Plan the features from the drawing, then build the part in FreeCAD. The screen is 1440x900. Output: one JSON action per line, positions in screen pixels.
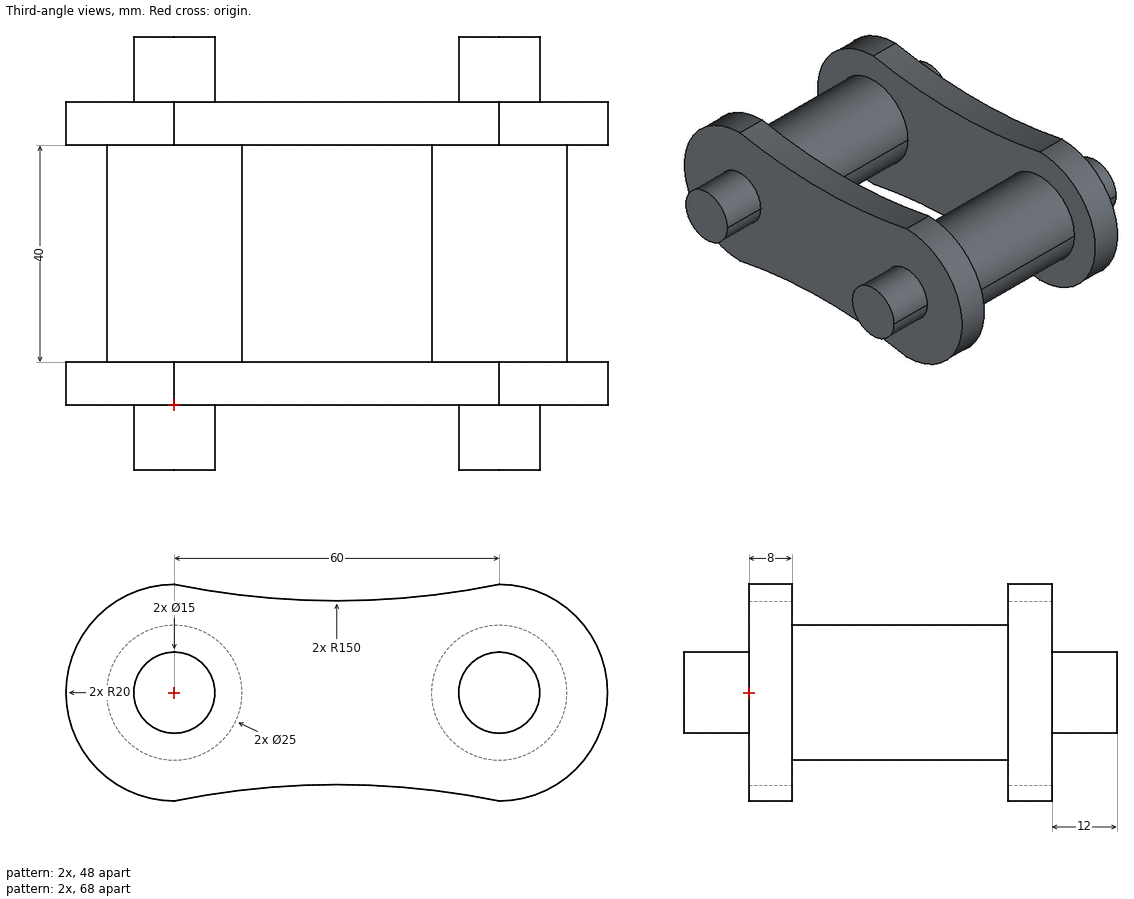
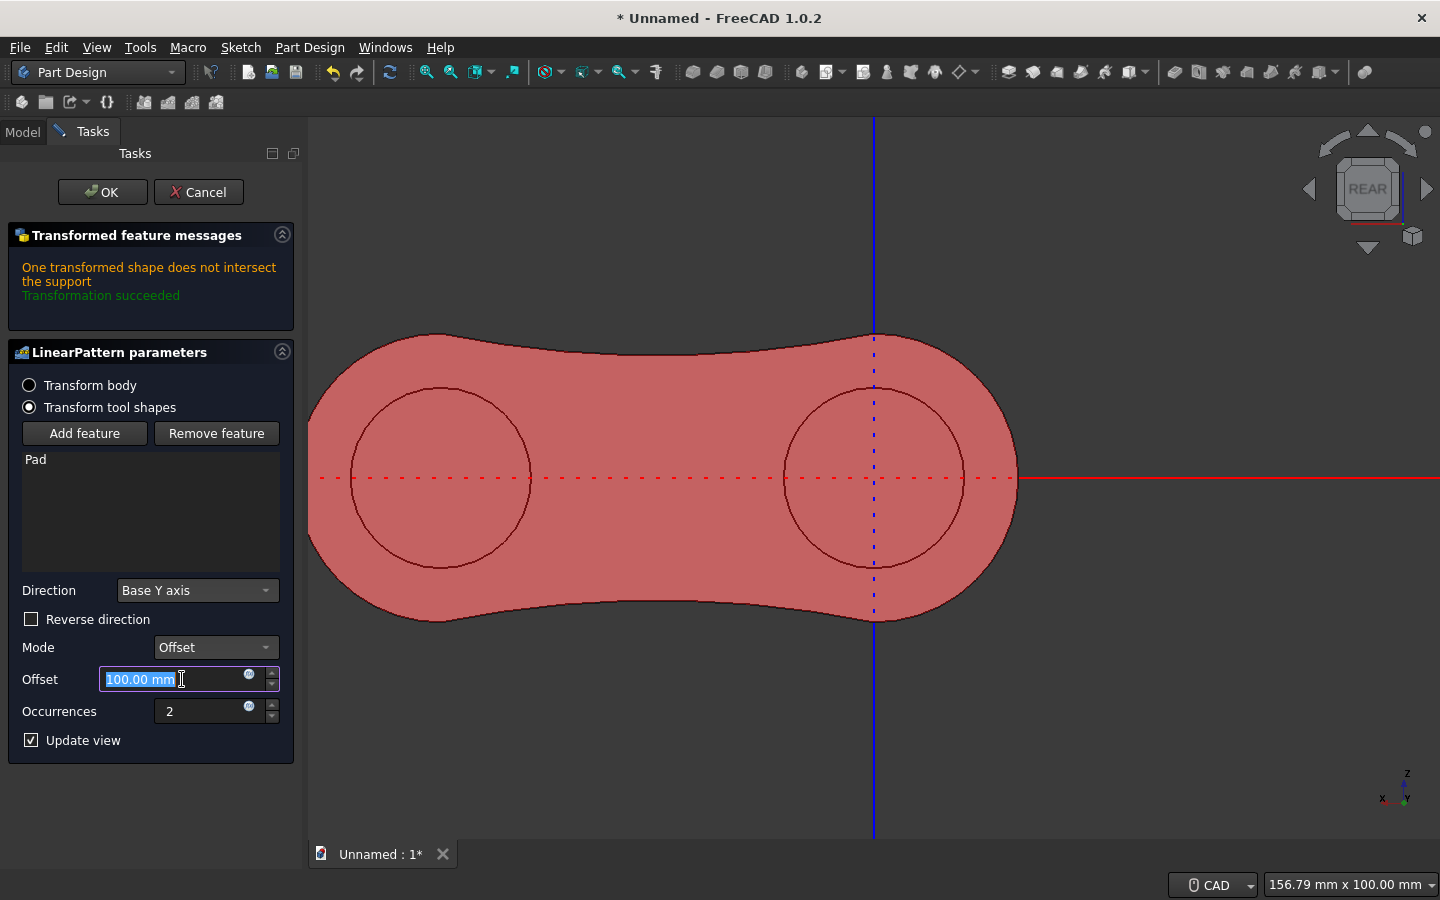
{"action": "type", "text": "48"}
{"action": "key", "text": "Tab"}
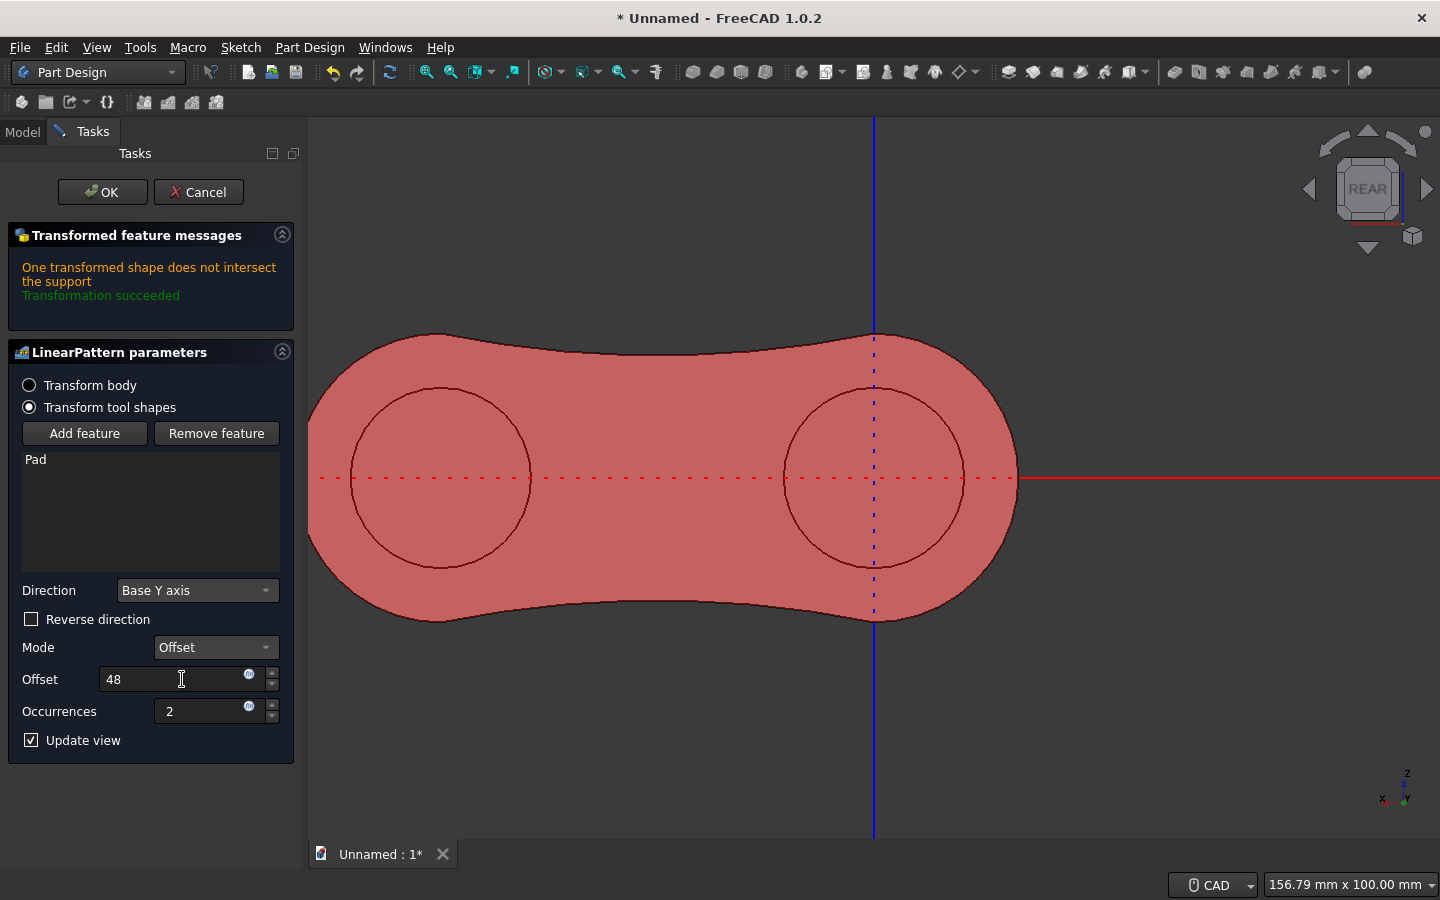
{"action": "triple_click", "coordinate": [209, 711]}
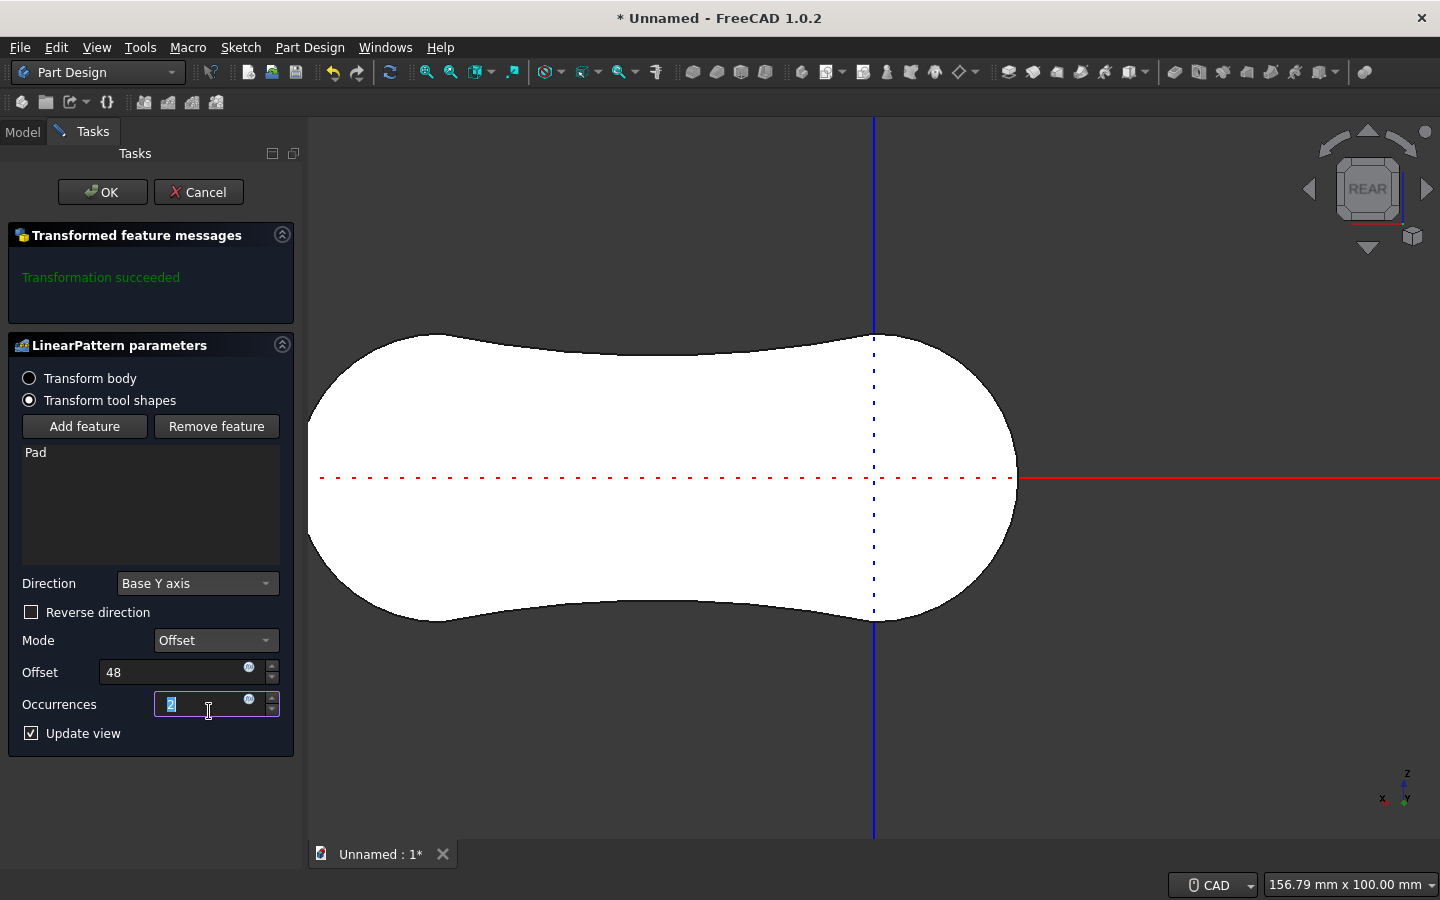
{"action": "type", "text": "2"}
{"action": "key", "text": "Tab"}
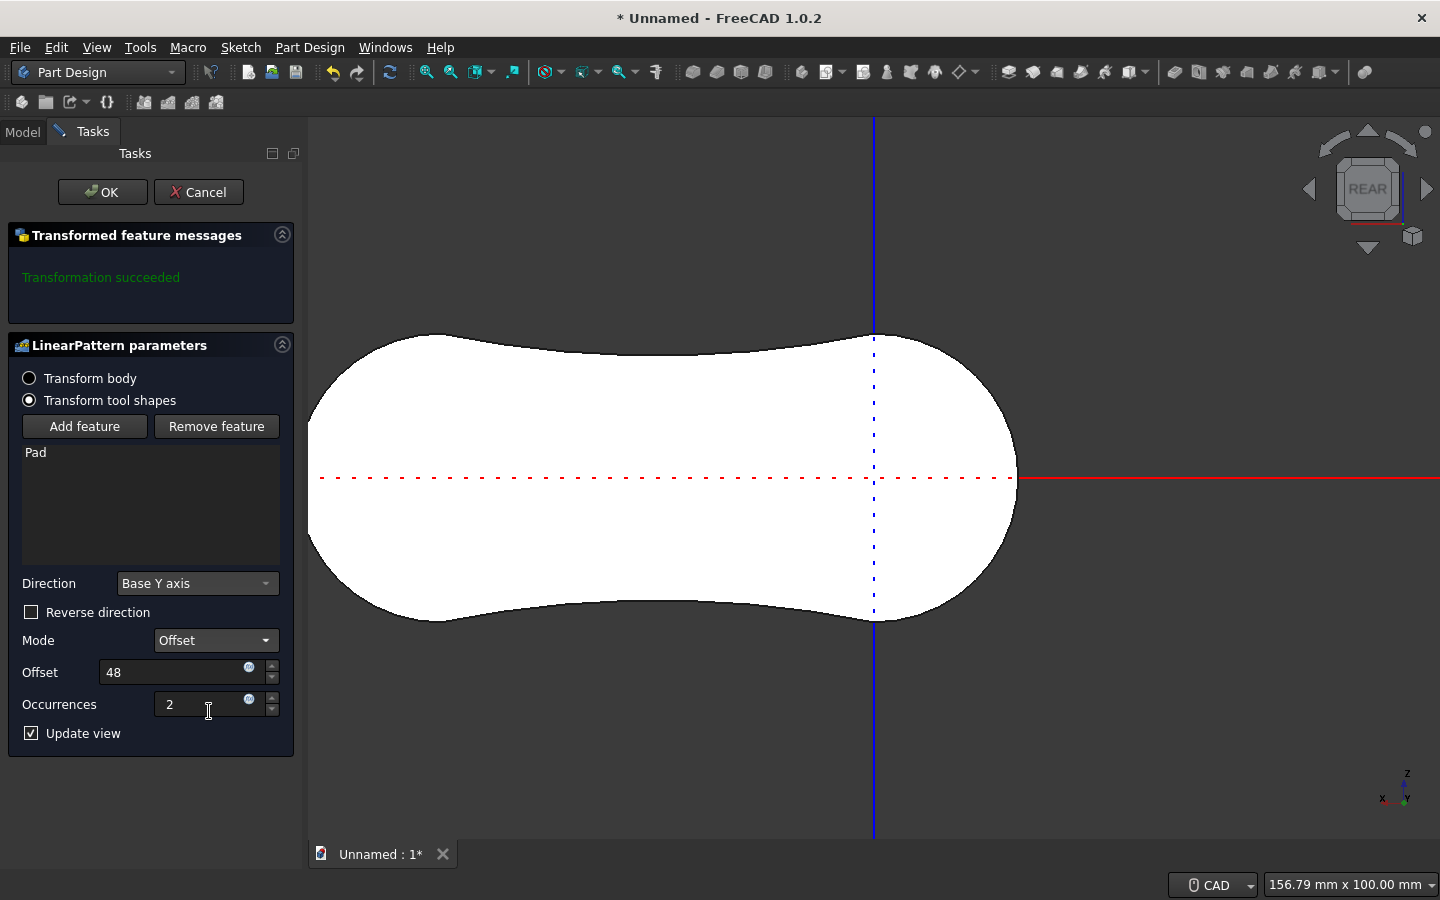
{"action": "left_click", "coordinate": [103, 192]}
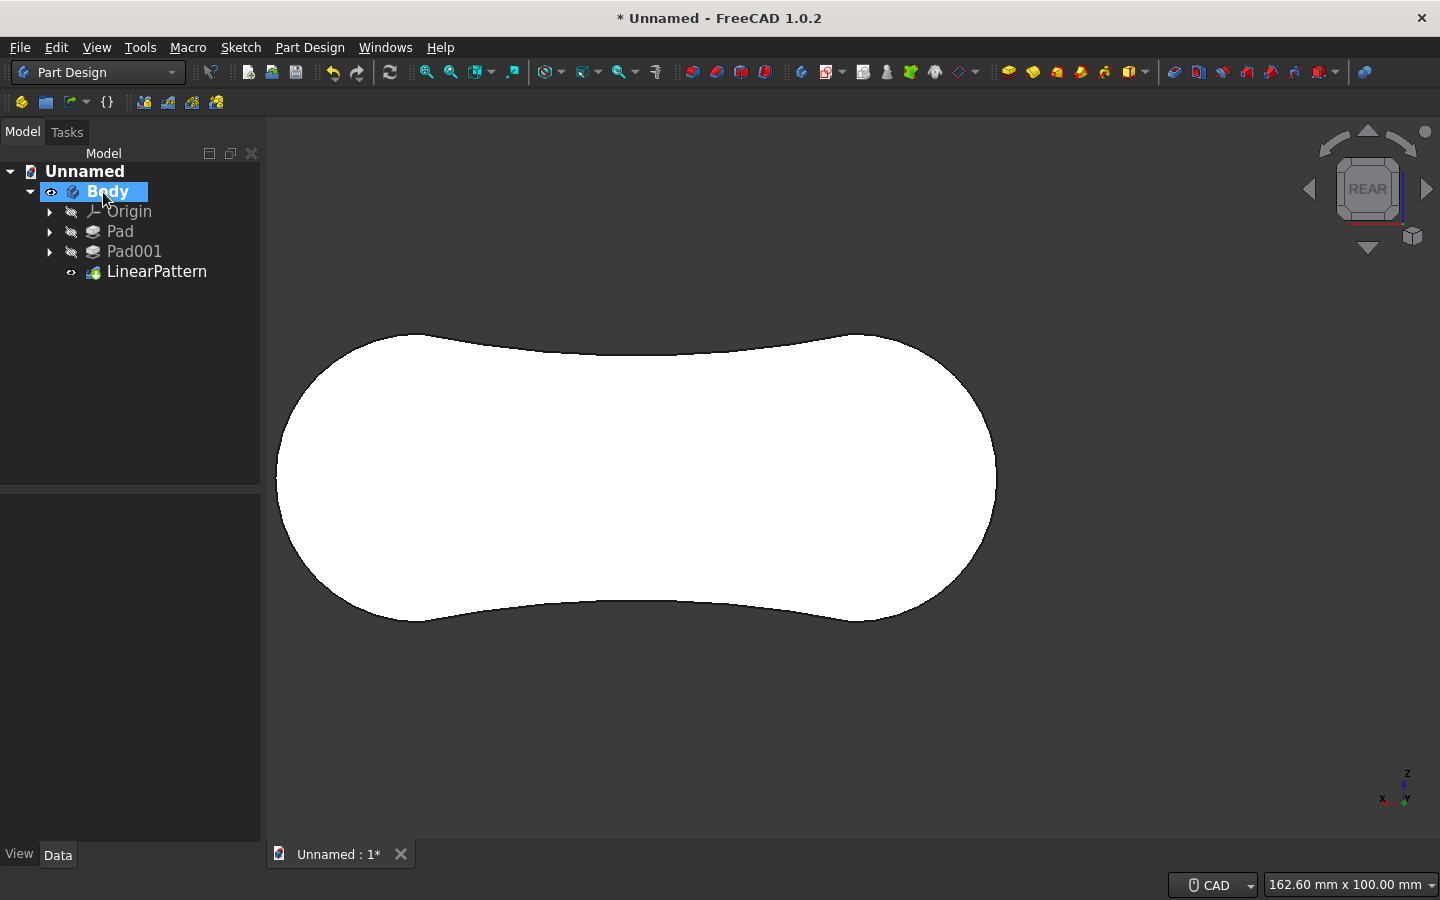
{"action": "left_click", "coordinate": [843, 477]}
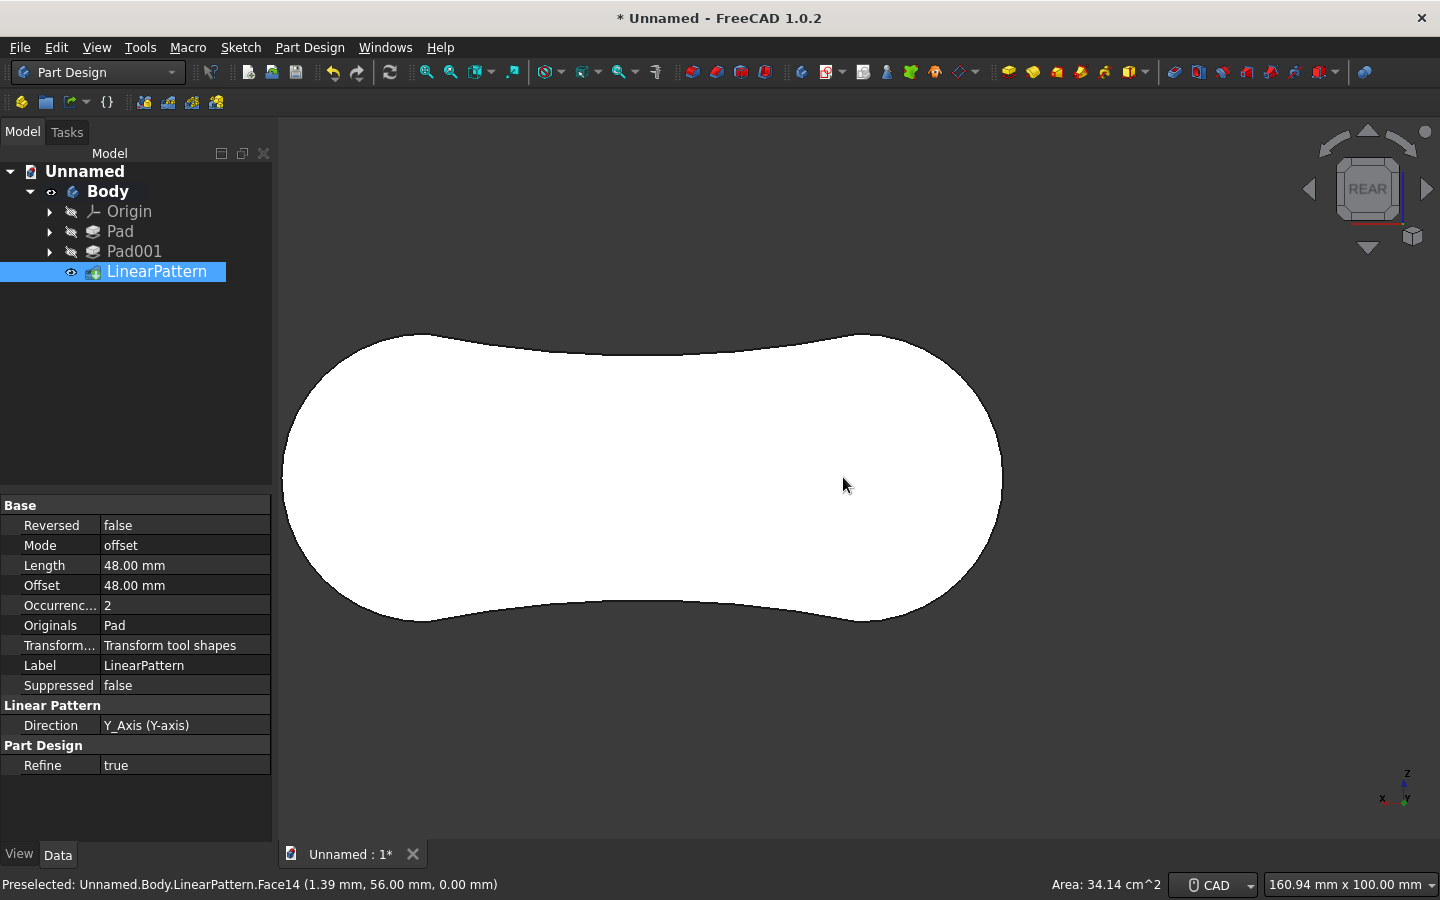
{"action": "left_click", "coordinate": [826, 72]}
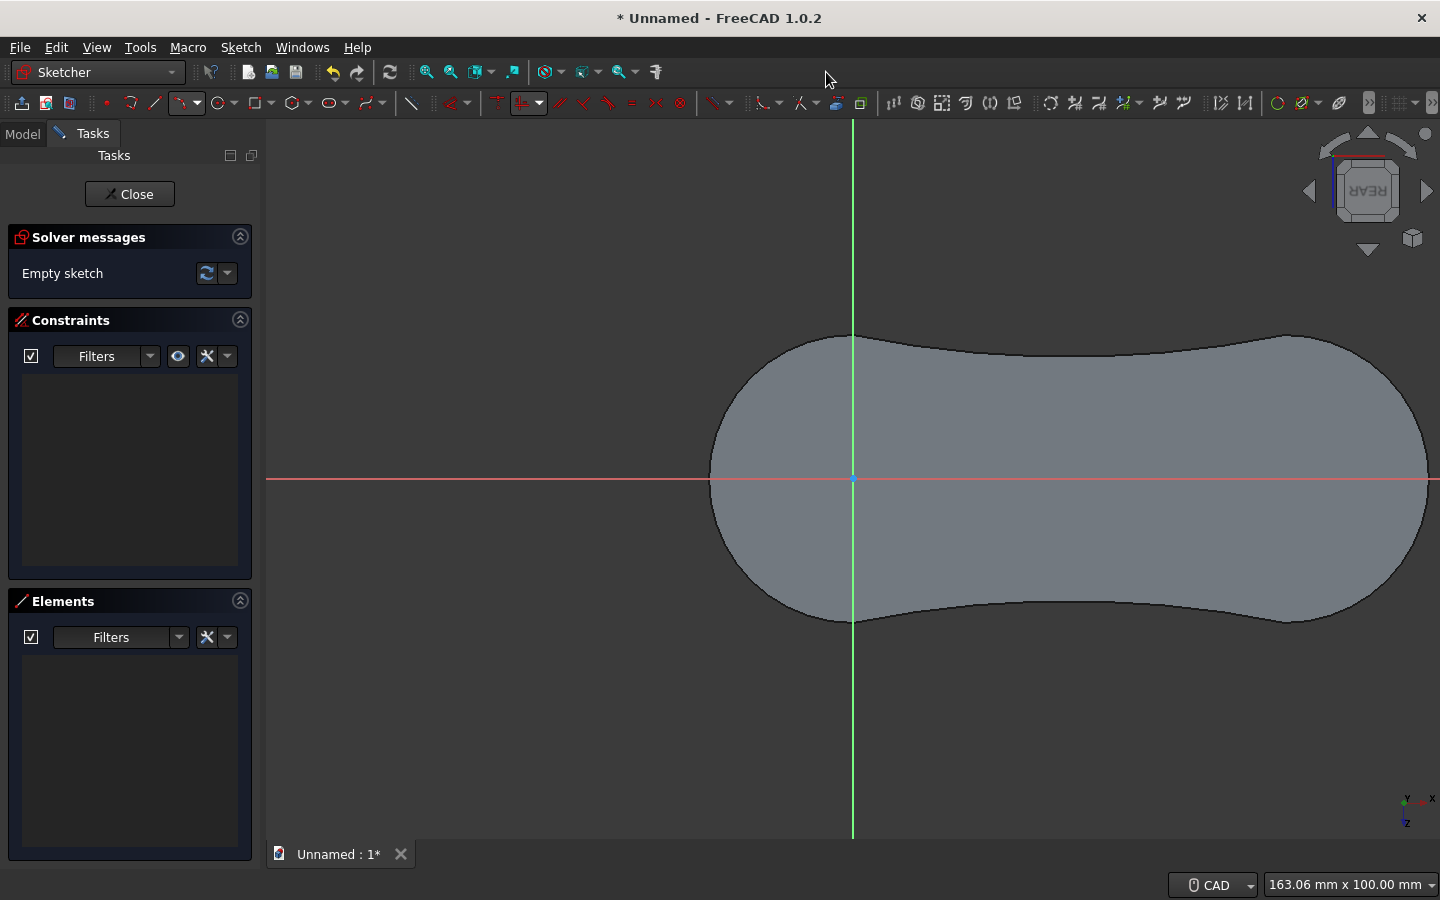
{"action": "scroll", "coordinate": [294, 479], "scroll_direction": "down", "scroll_amount": 1}